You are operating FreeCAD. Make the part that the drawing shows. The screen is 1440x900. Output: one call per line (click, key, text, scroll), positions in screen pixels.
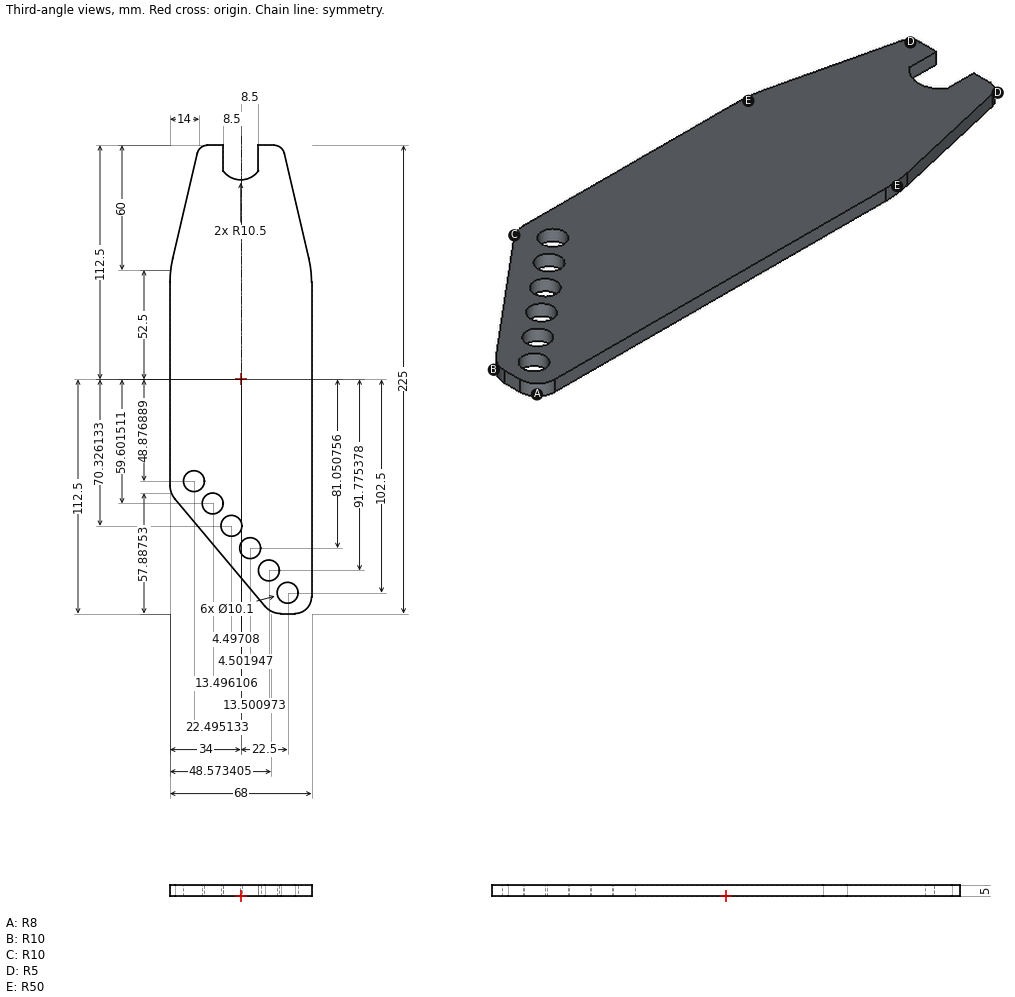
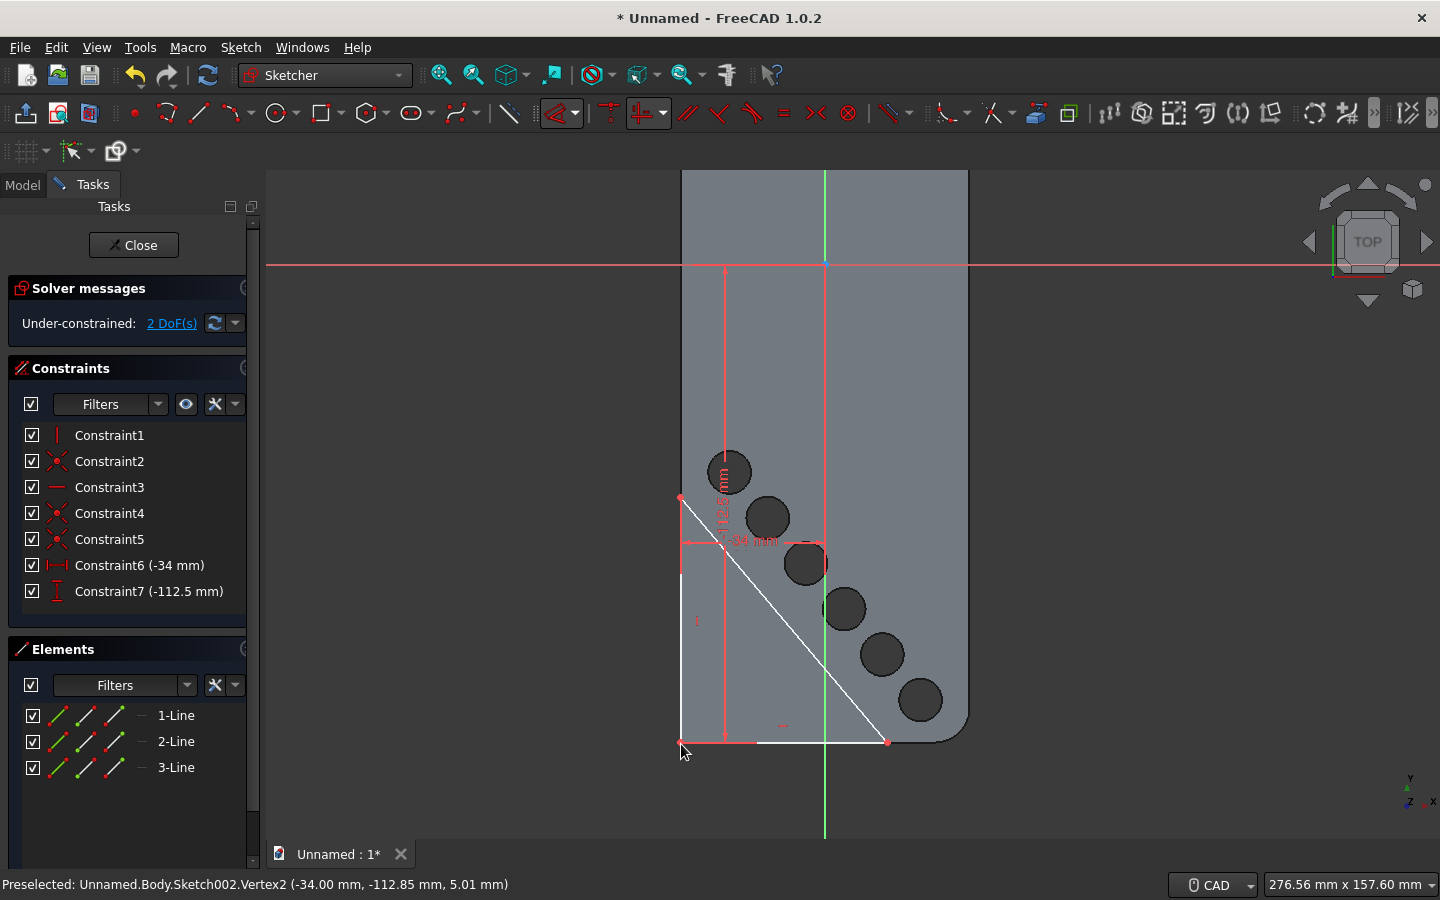
click(681, 571)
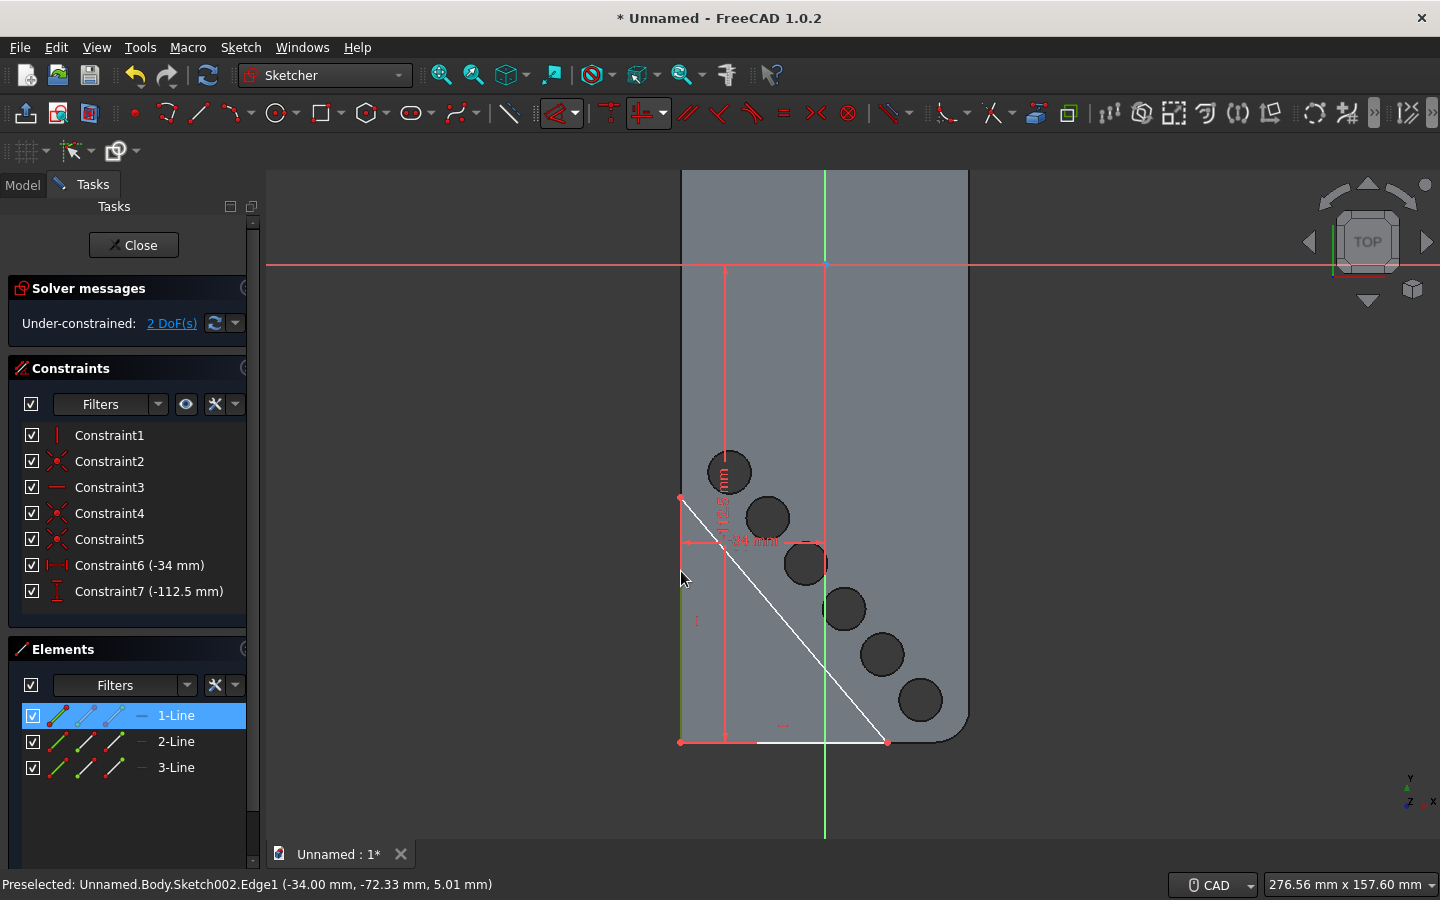
key(i)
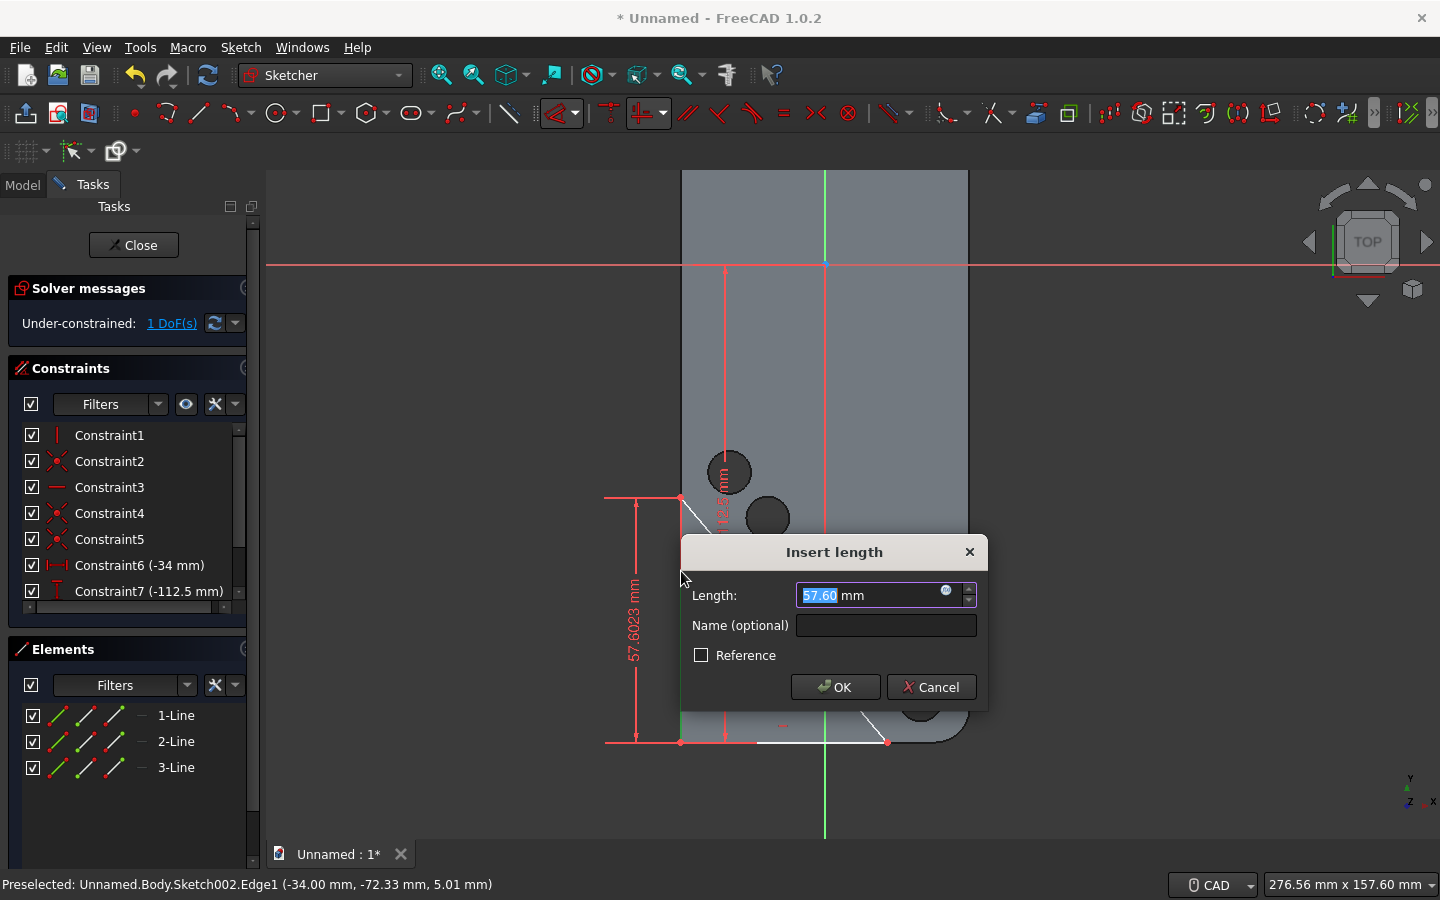
text(57.88753)
key(Return)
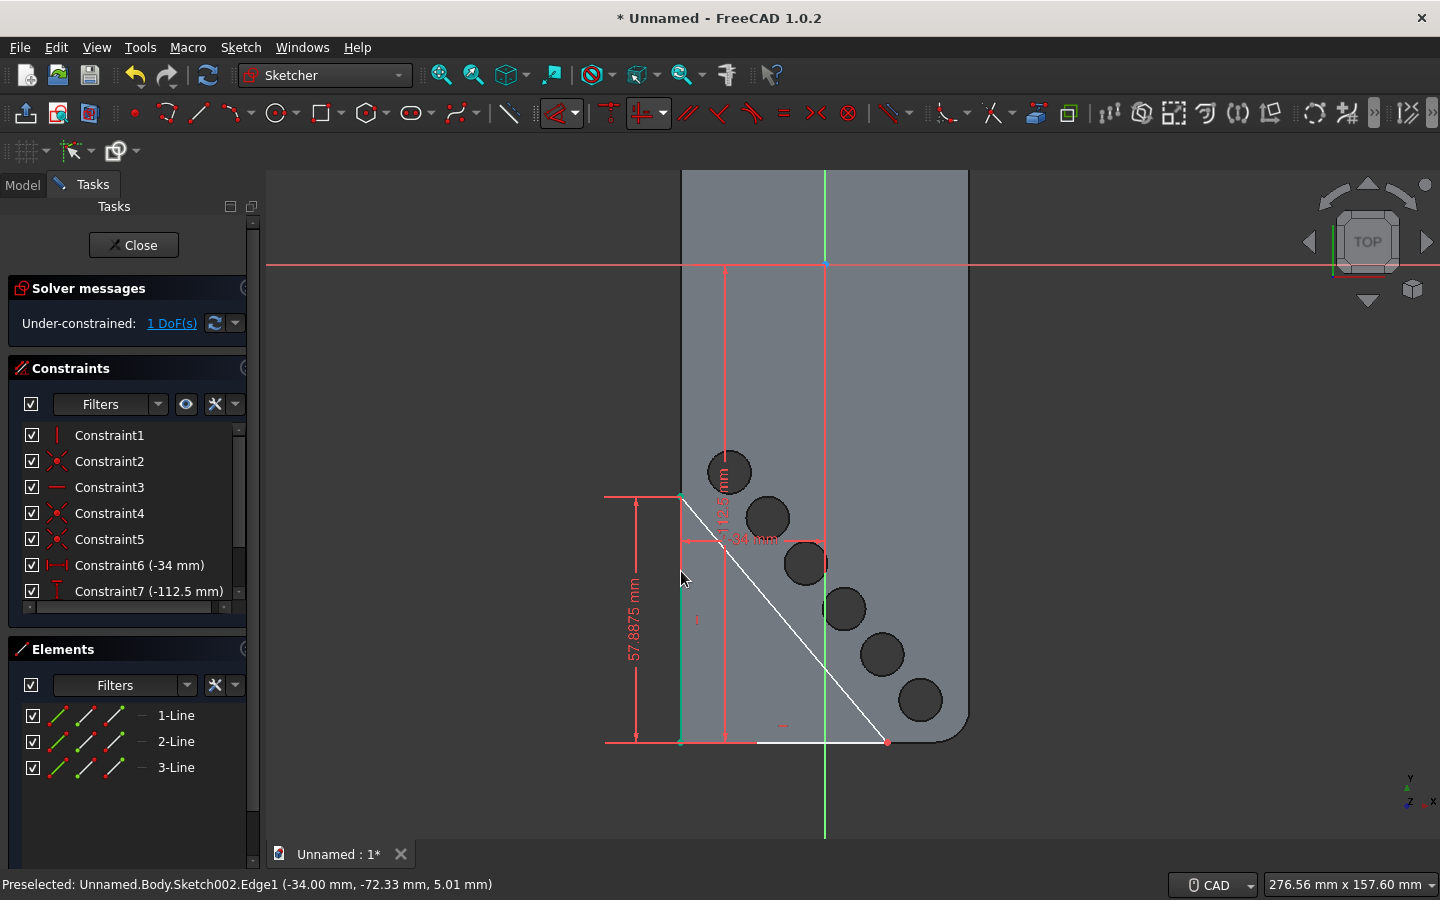
click(743, 743)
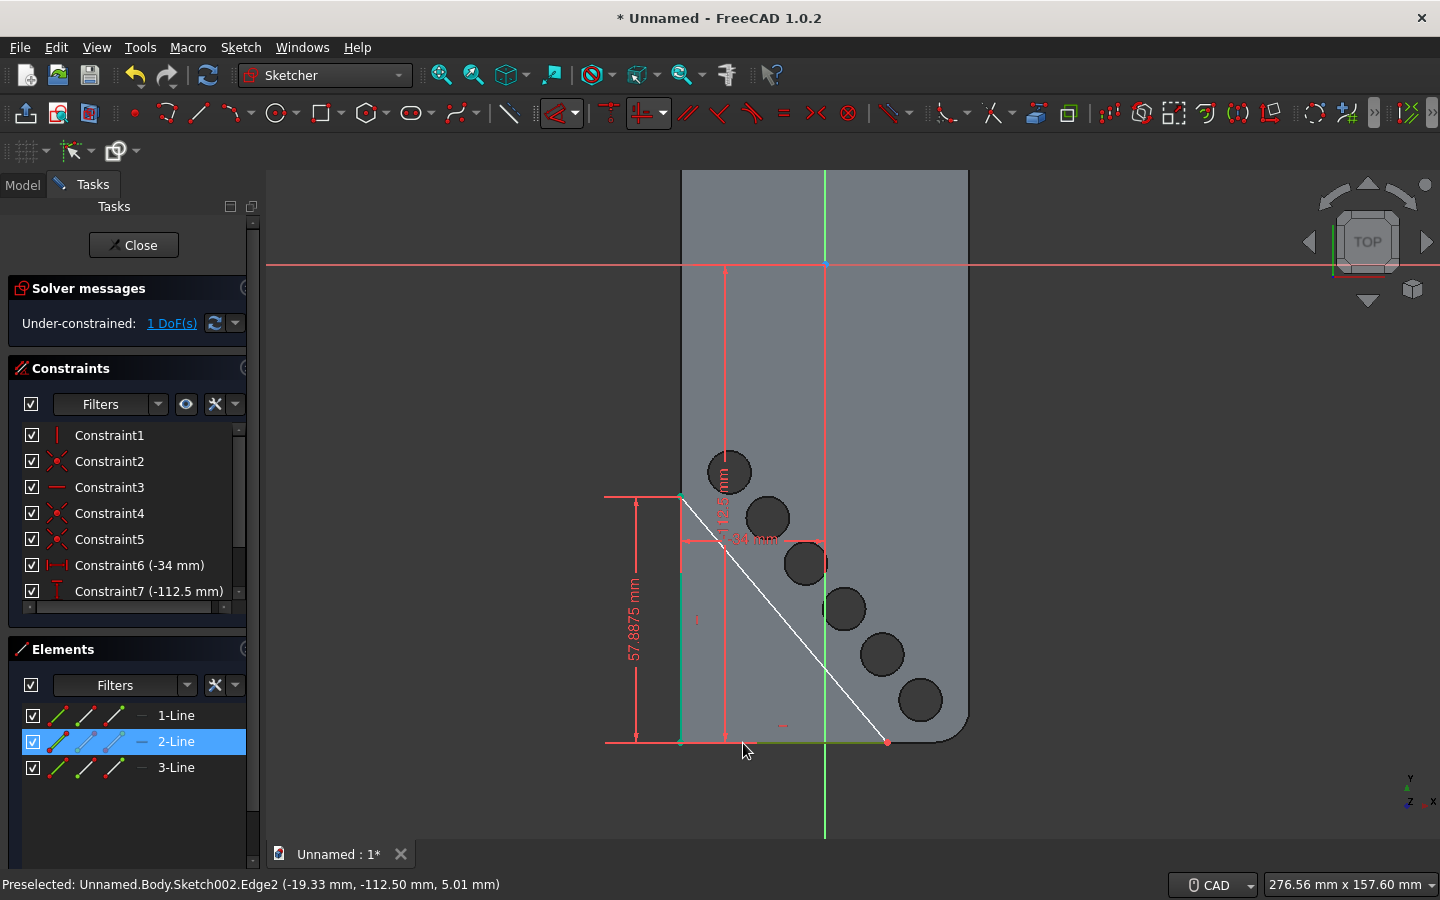
key(l)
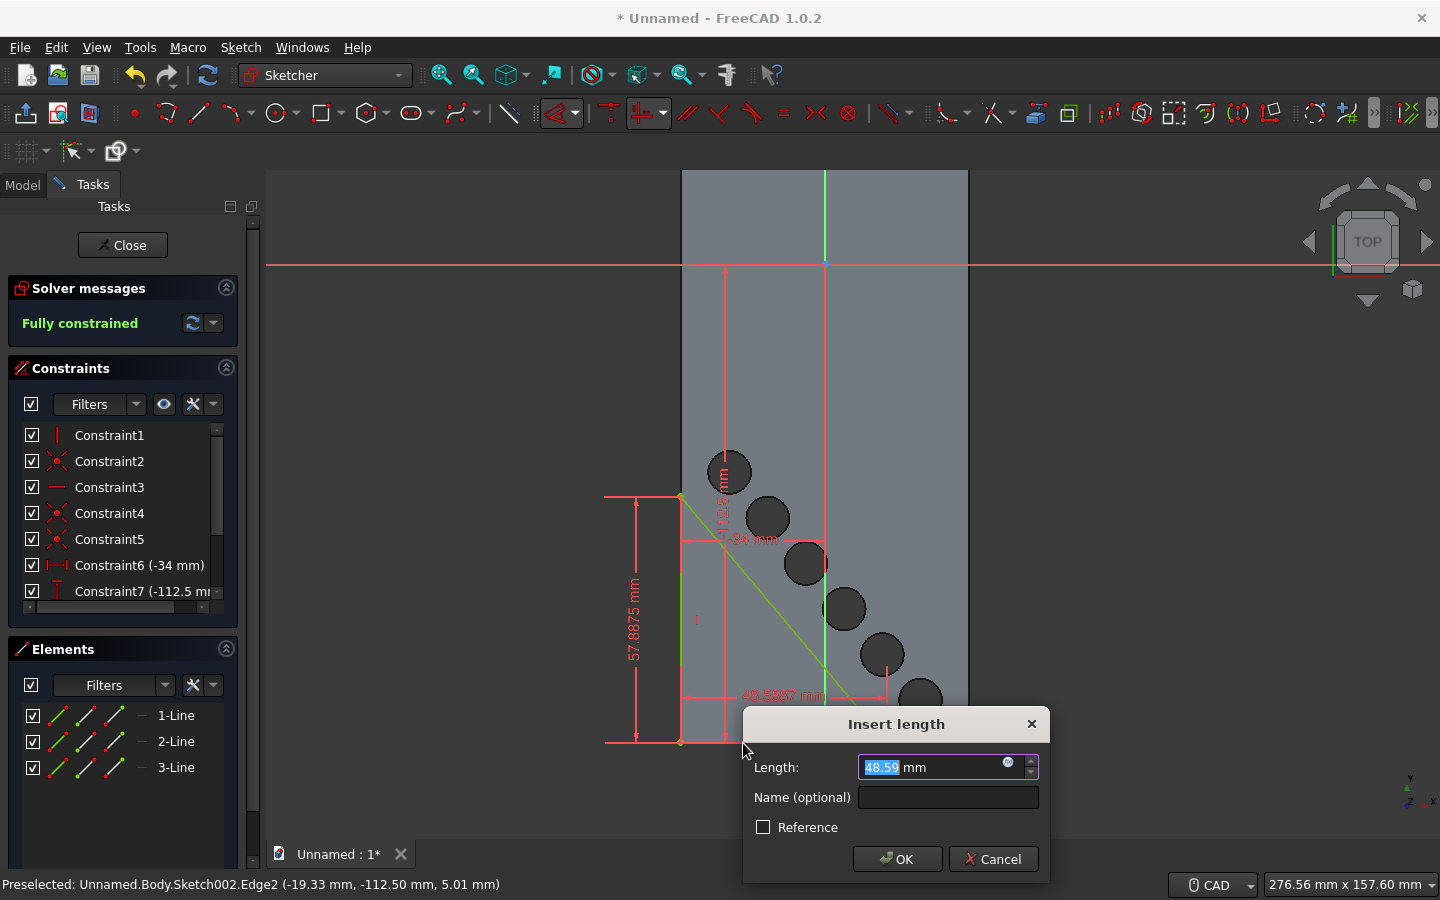
text(48.573405)
key(Return)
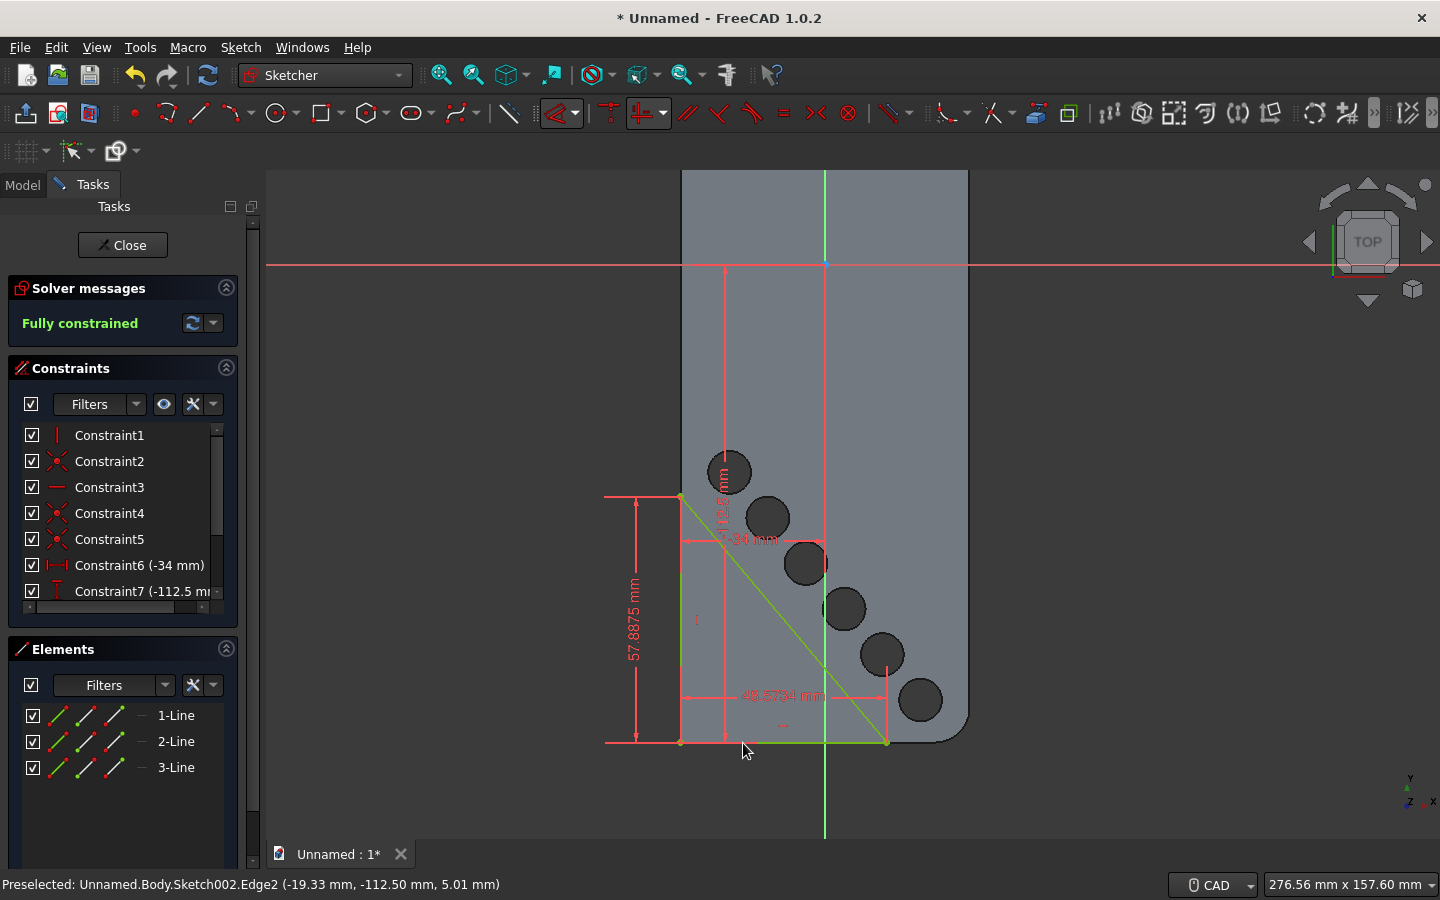
click(123, 245)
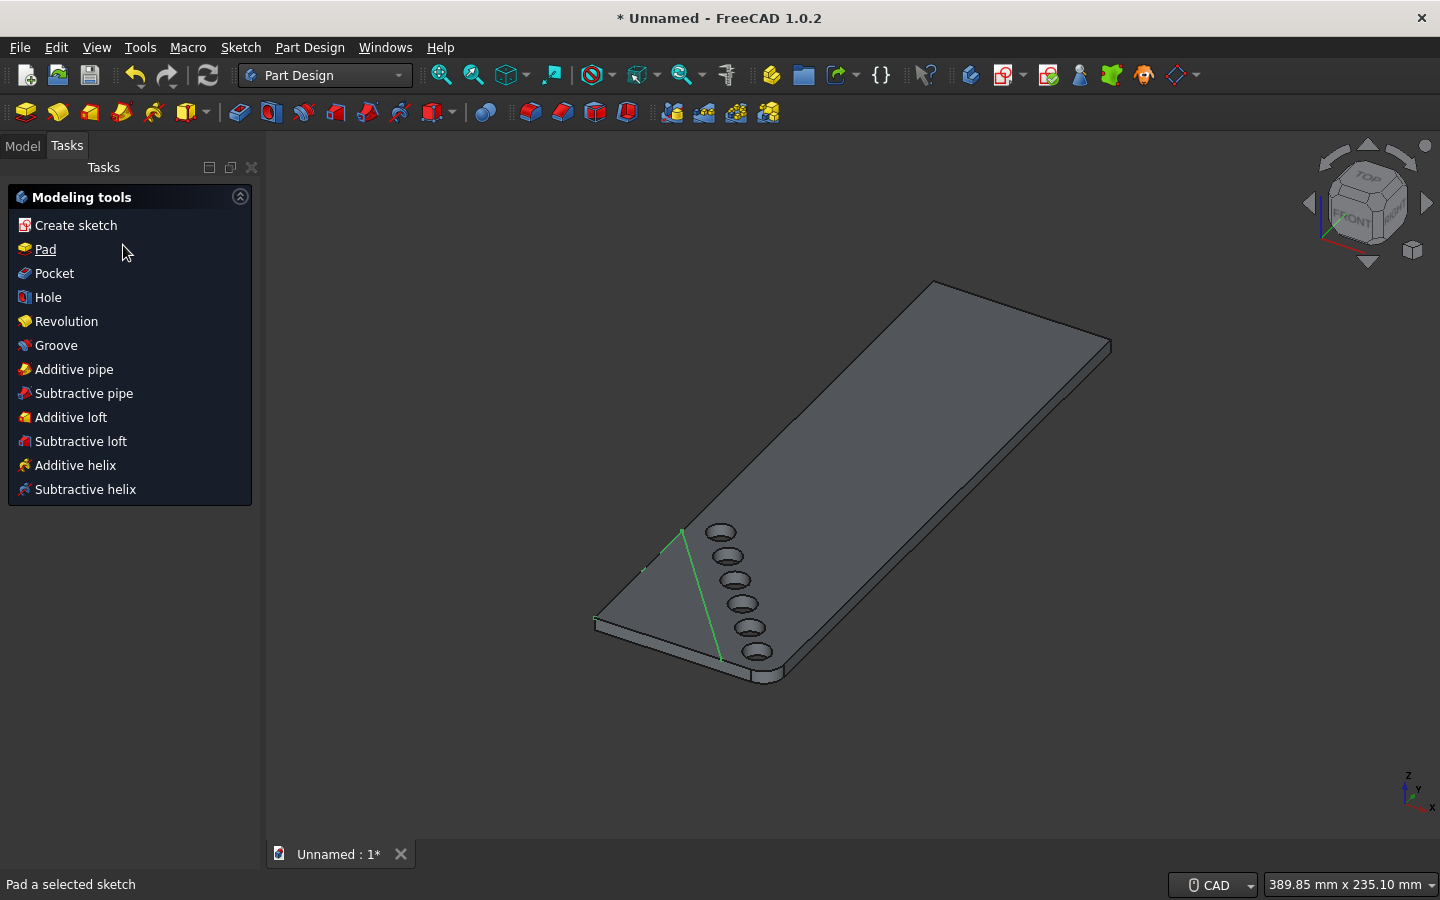
click(240, 112)